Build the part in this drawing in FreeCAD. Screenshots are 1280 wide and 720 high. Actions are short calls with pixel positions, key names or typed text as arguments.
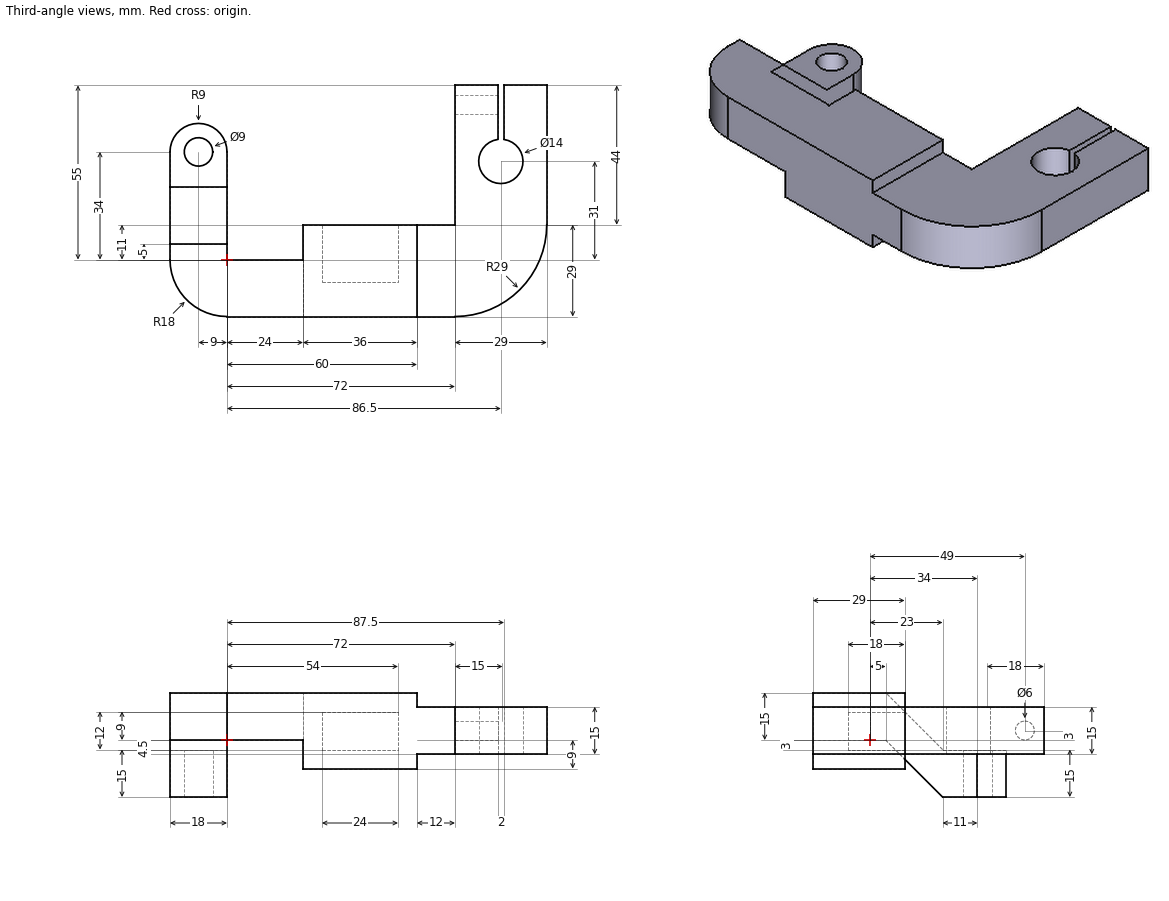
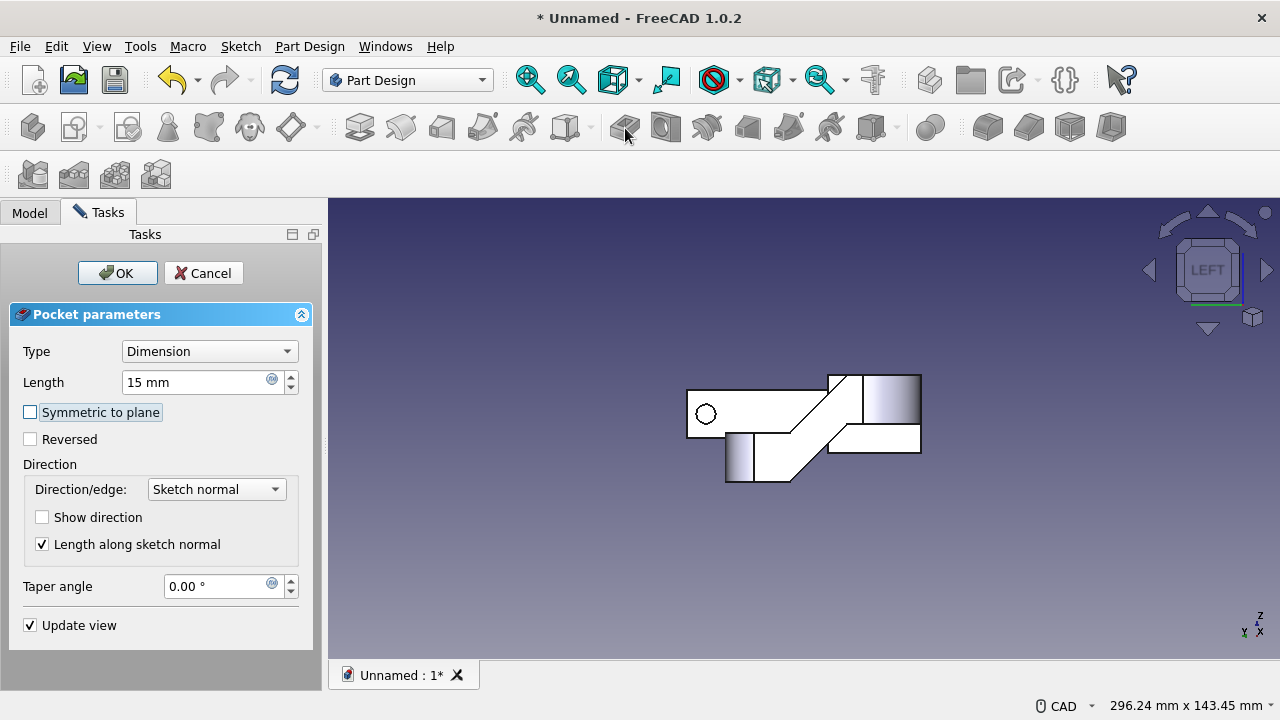
click(118, 273)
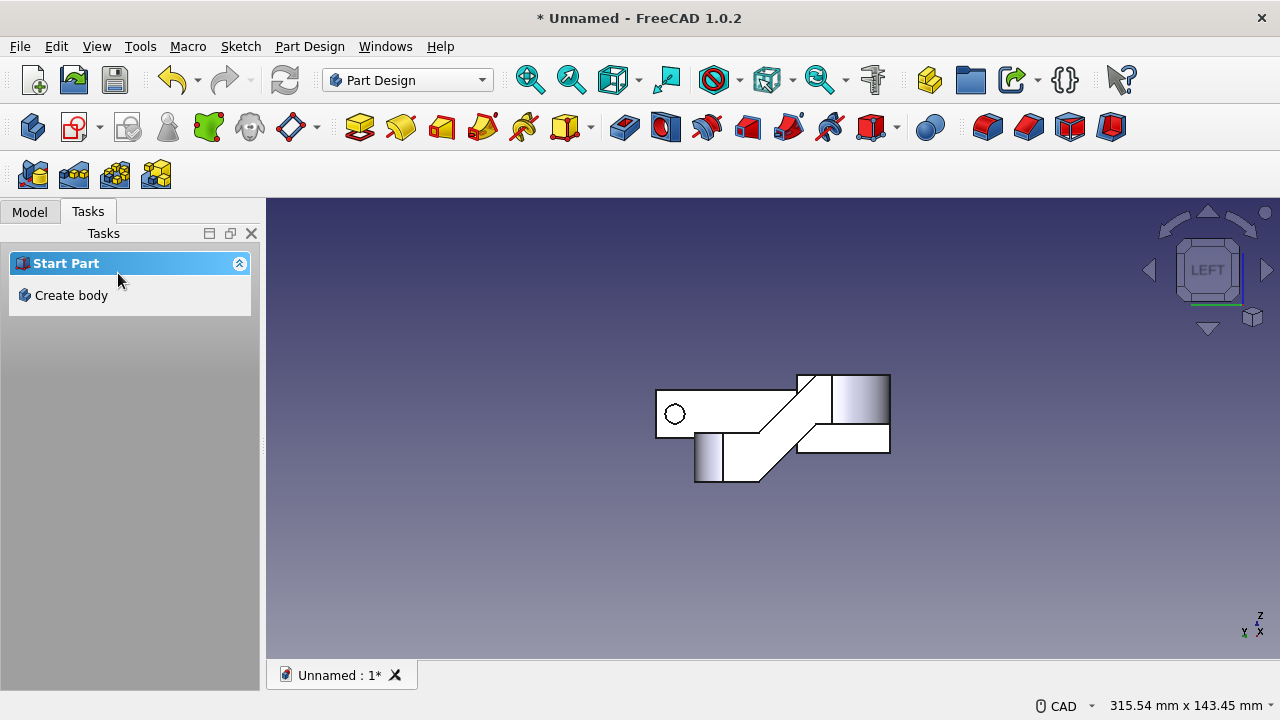
click(531, 80)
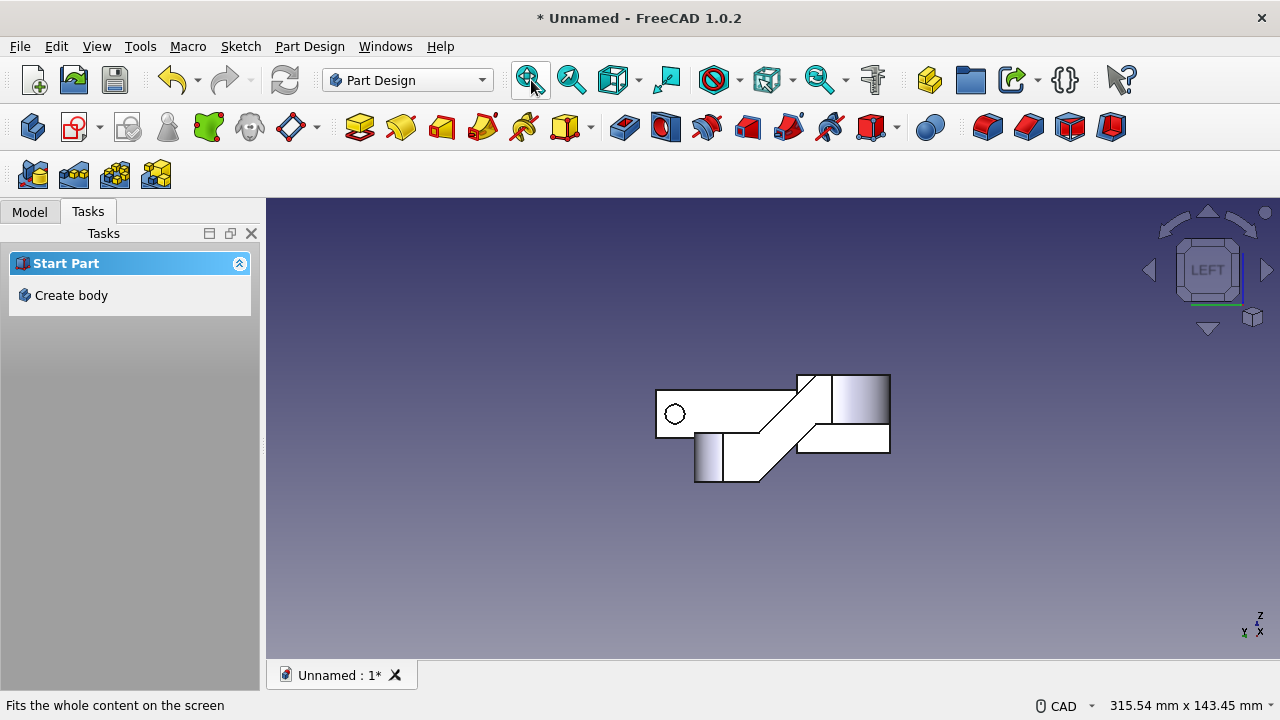
key(4)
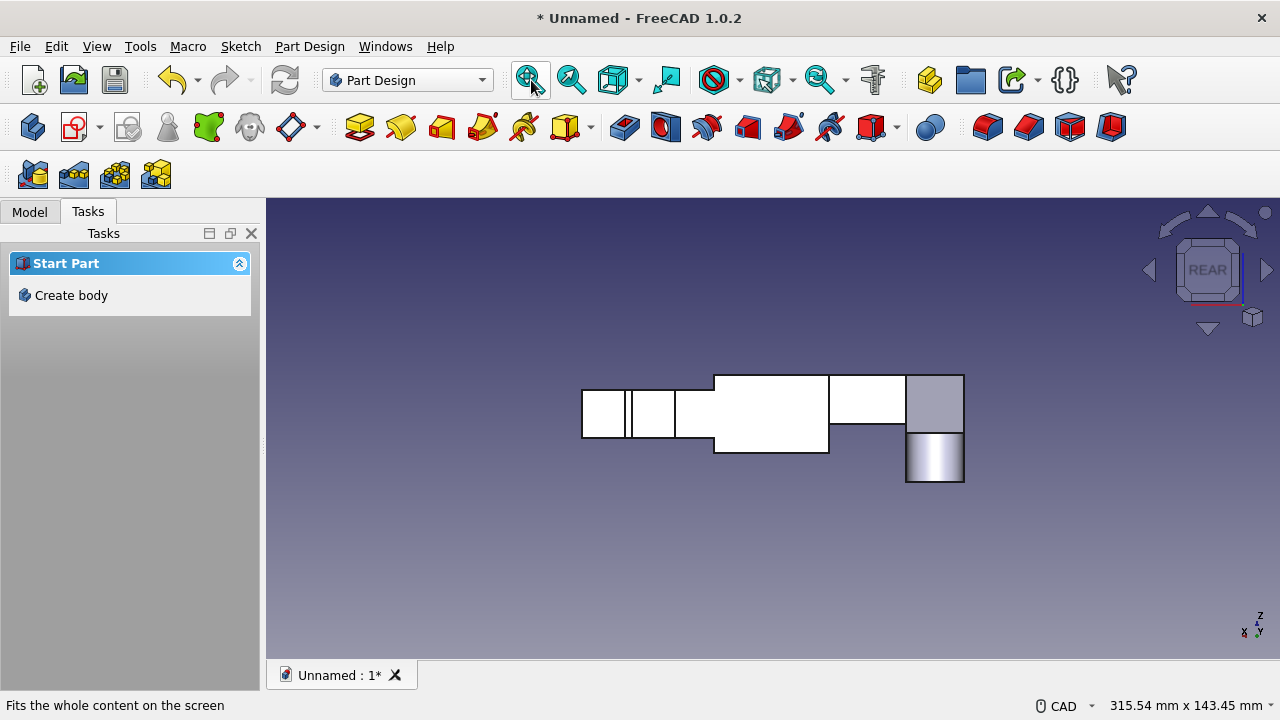
click(531, 80)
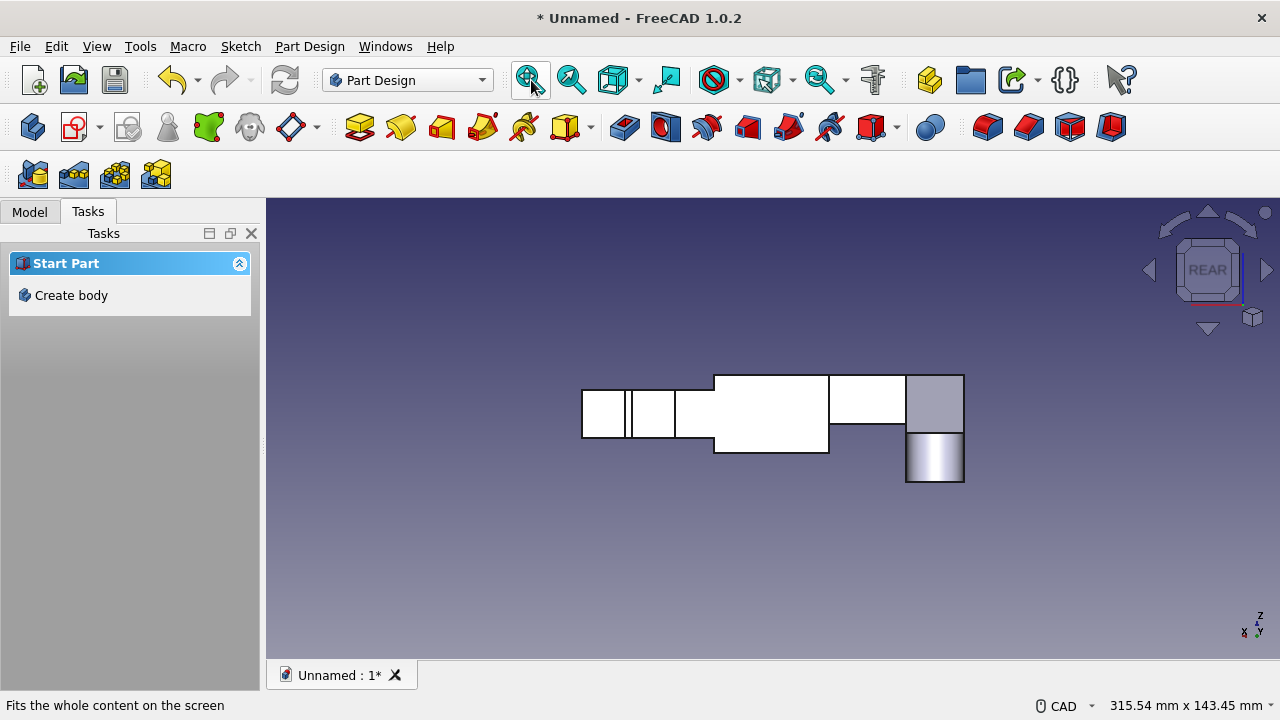
click(752, 413)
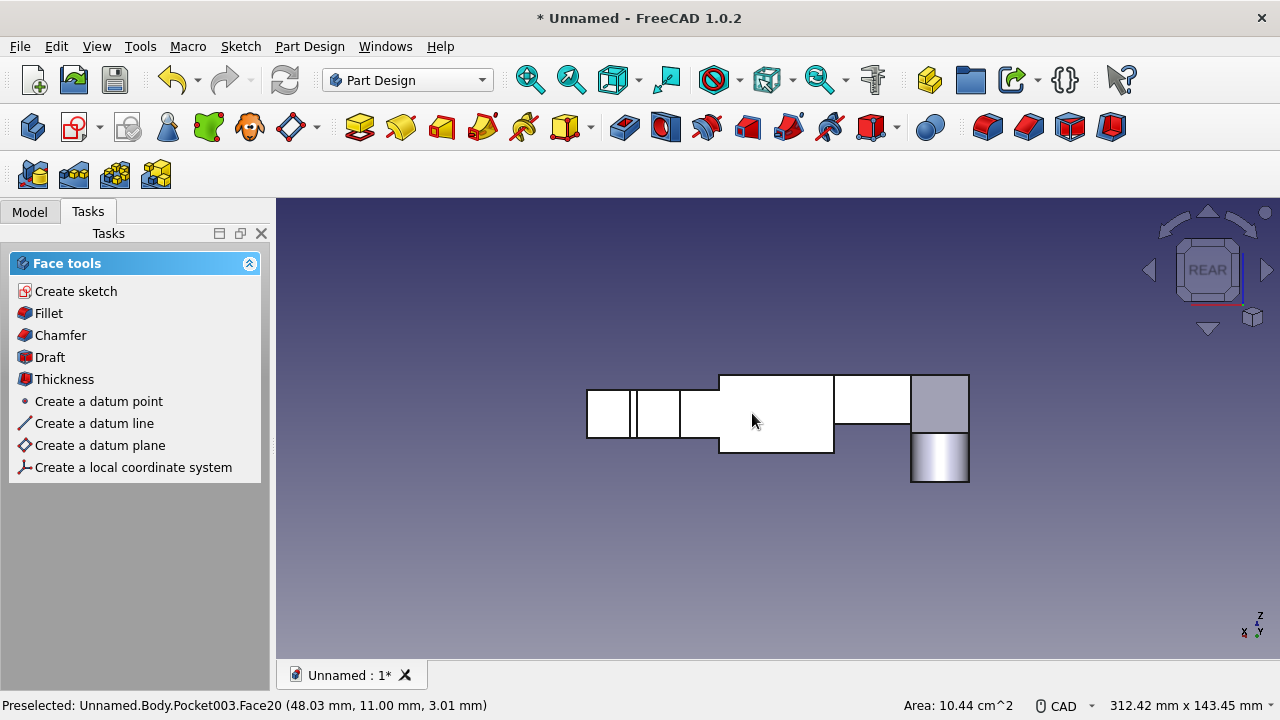
click(74, 128)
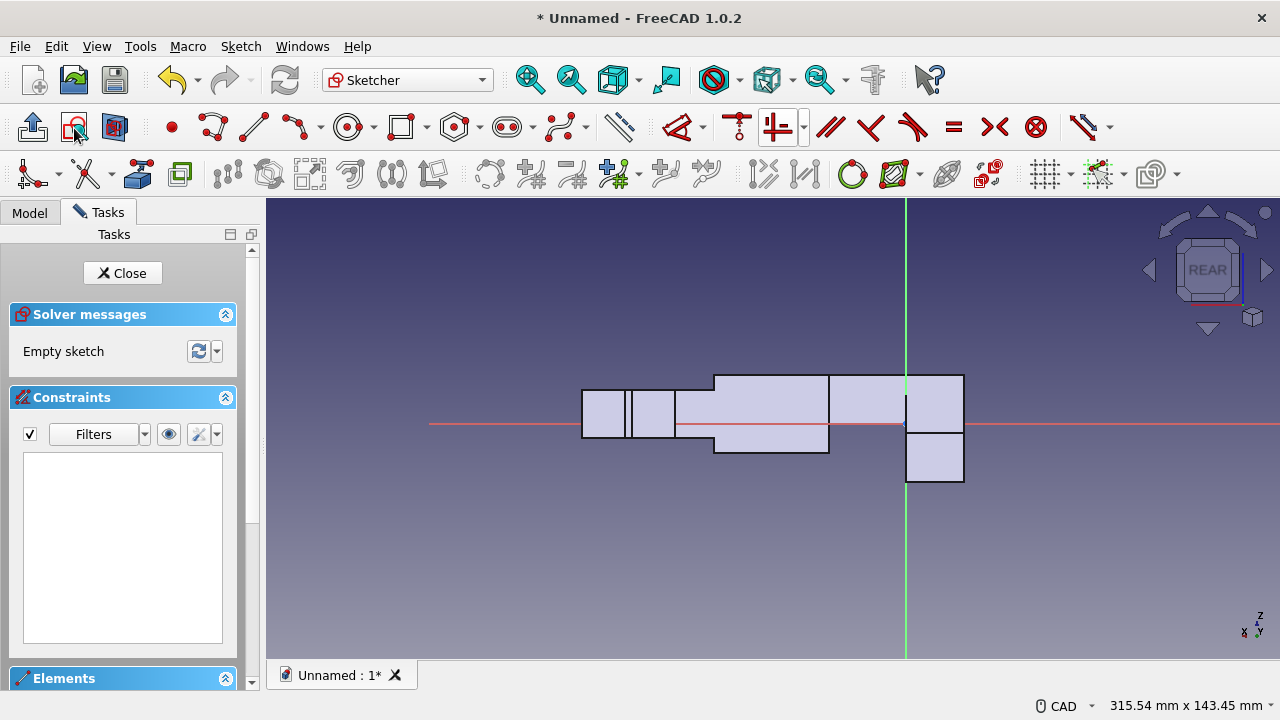
click(115, 128)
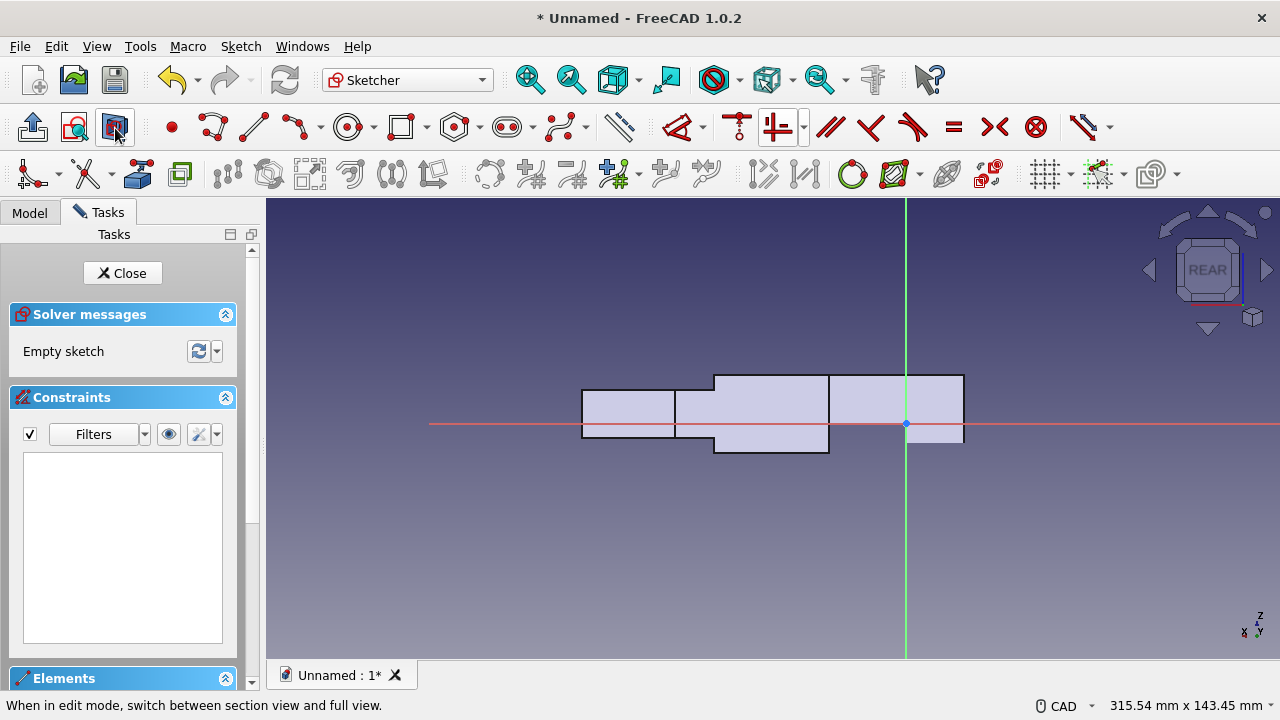
scroll(869, 408, up, 6)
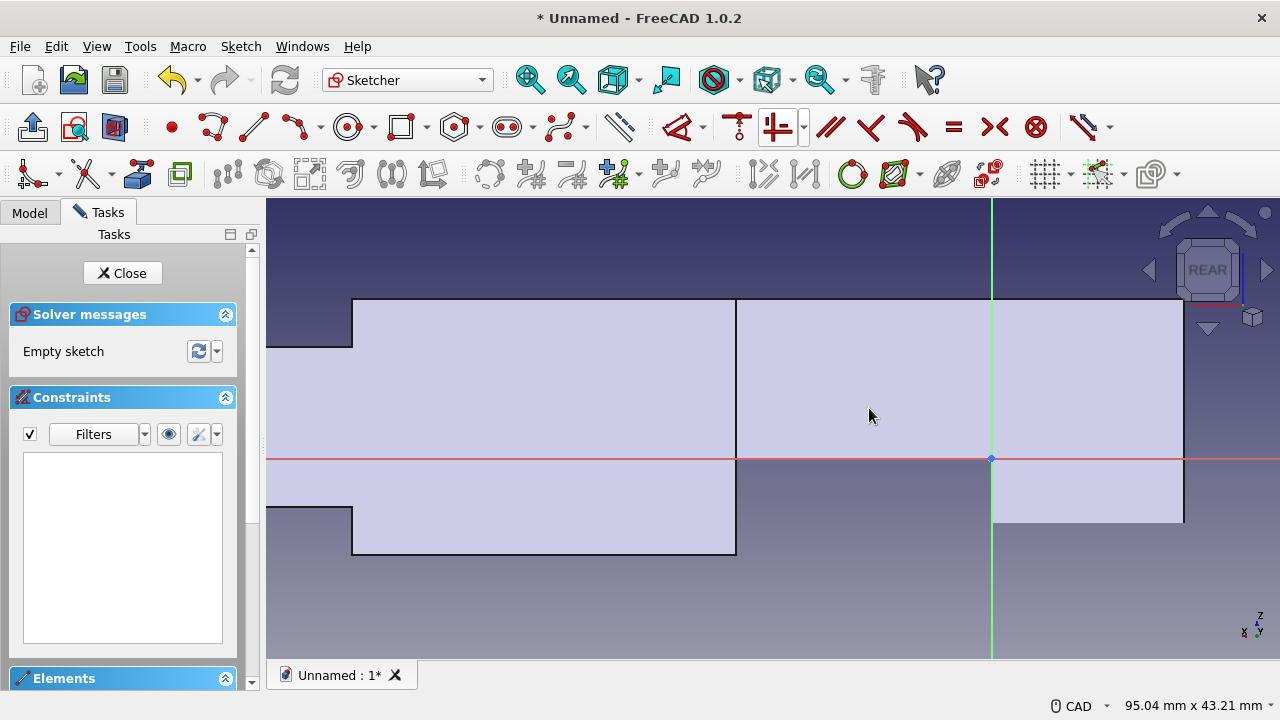
click(400, 128)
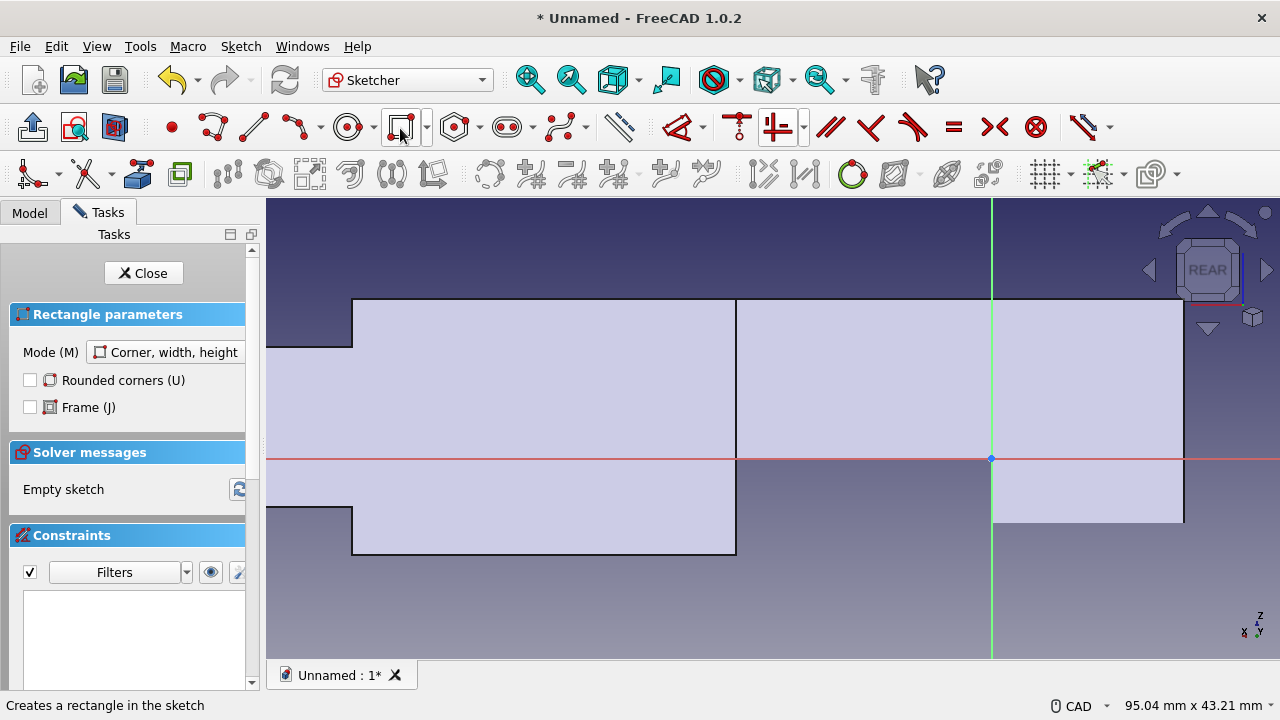
click(416, 363)
move(672, 491)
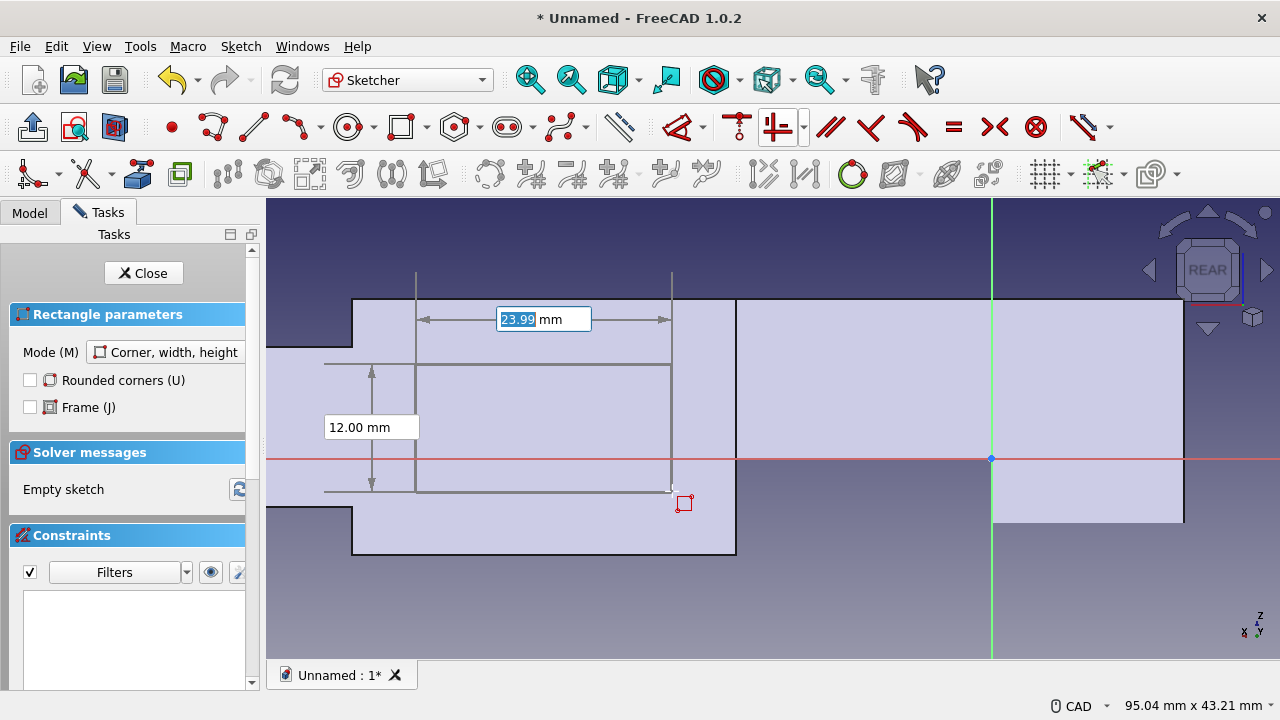
text(24)
key(Tab)
text(12)
key(Return)
key(Escape)